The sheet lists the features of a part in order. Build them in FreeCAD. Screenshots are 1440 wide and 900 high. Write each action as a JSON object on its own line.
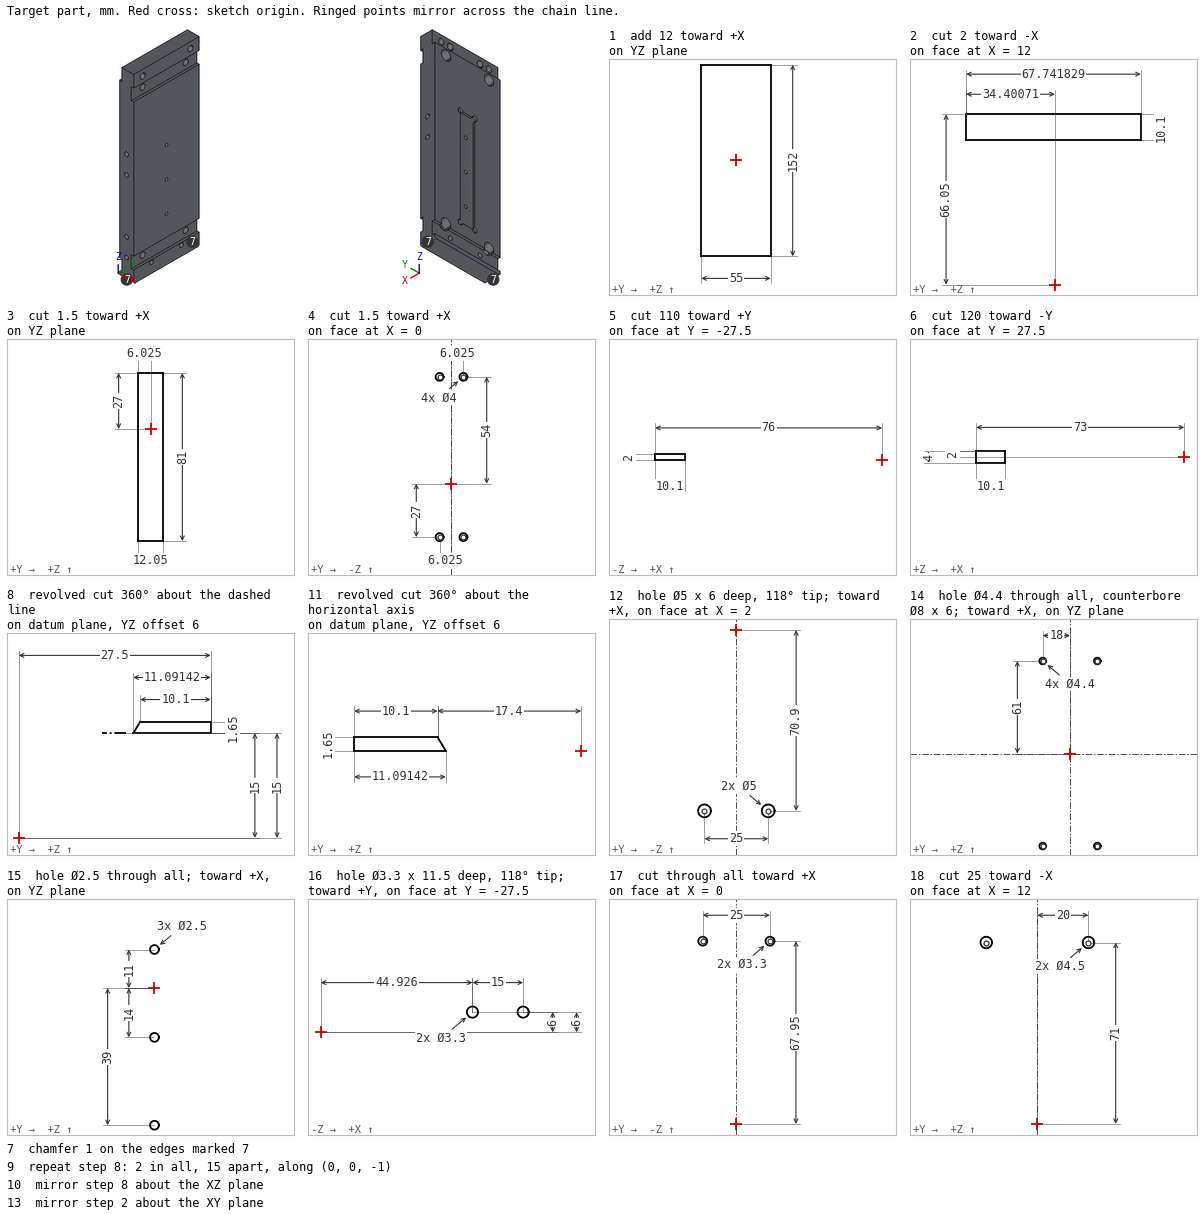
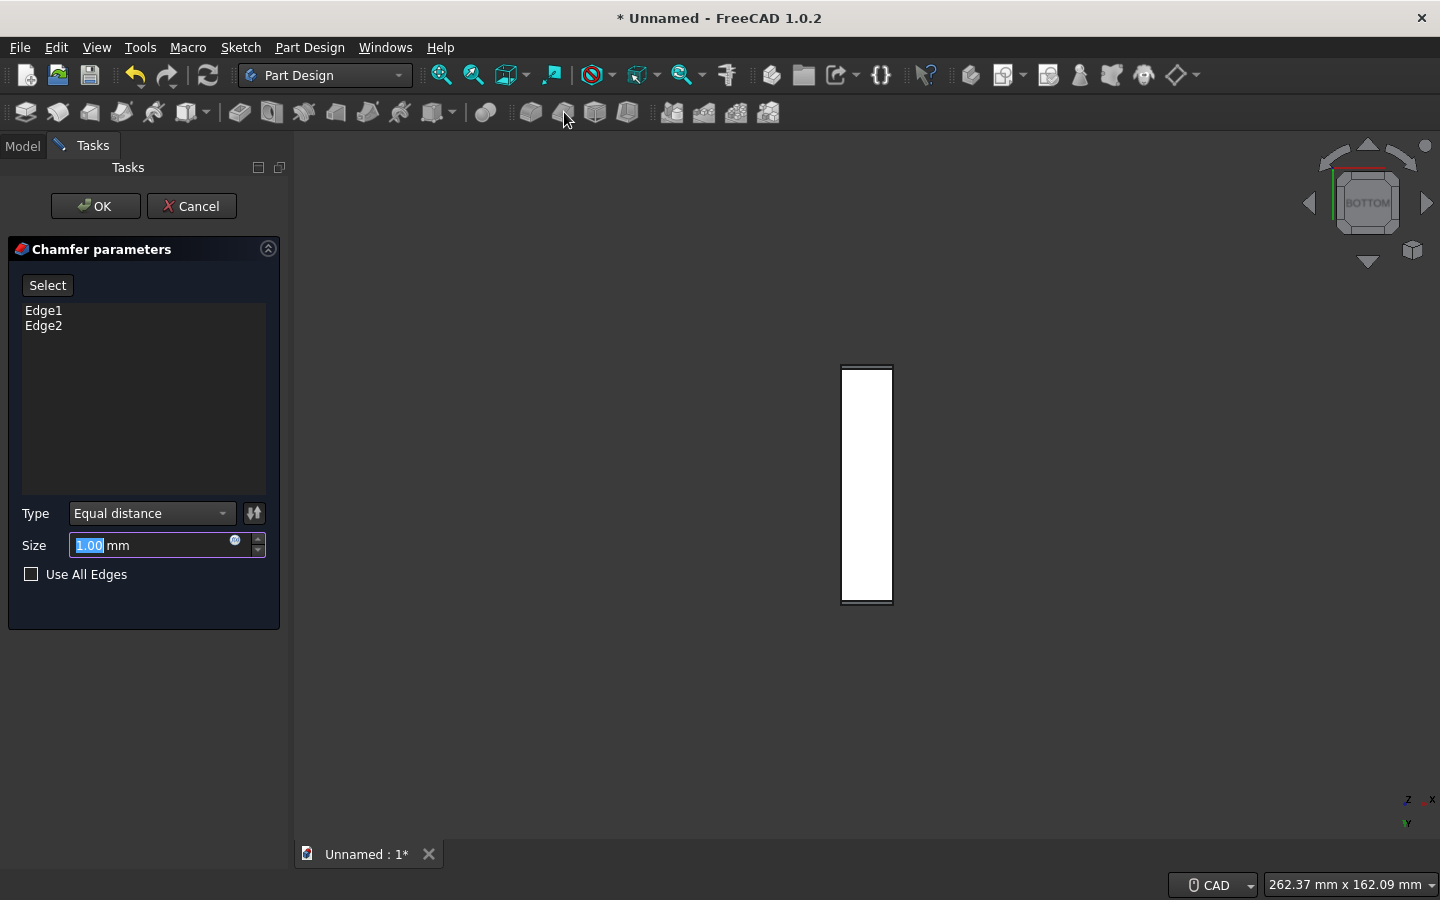
{"action": "type", "text": "1"}
{"action": "key", "text": "Tab"}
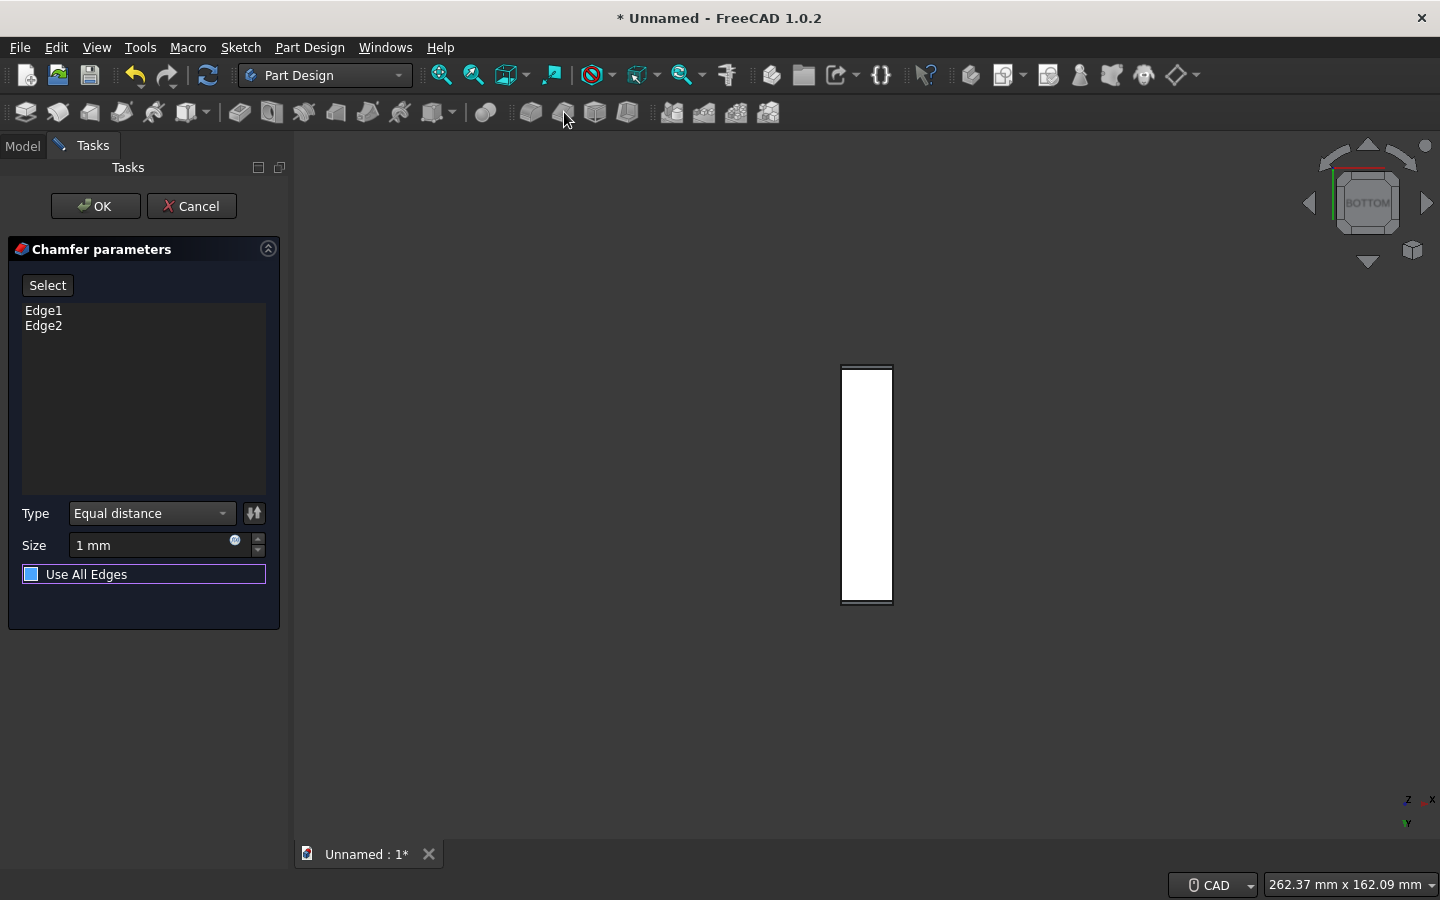
{"action": "left_click", "coordinate": [96, 206]}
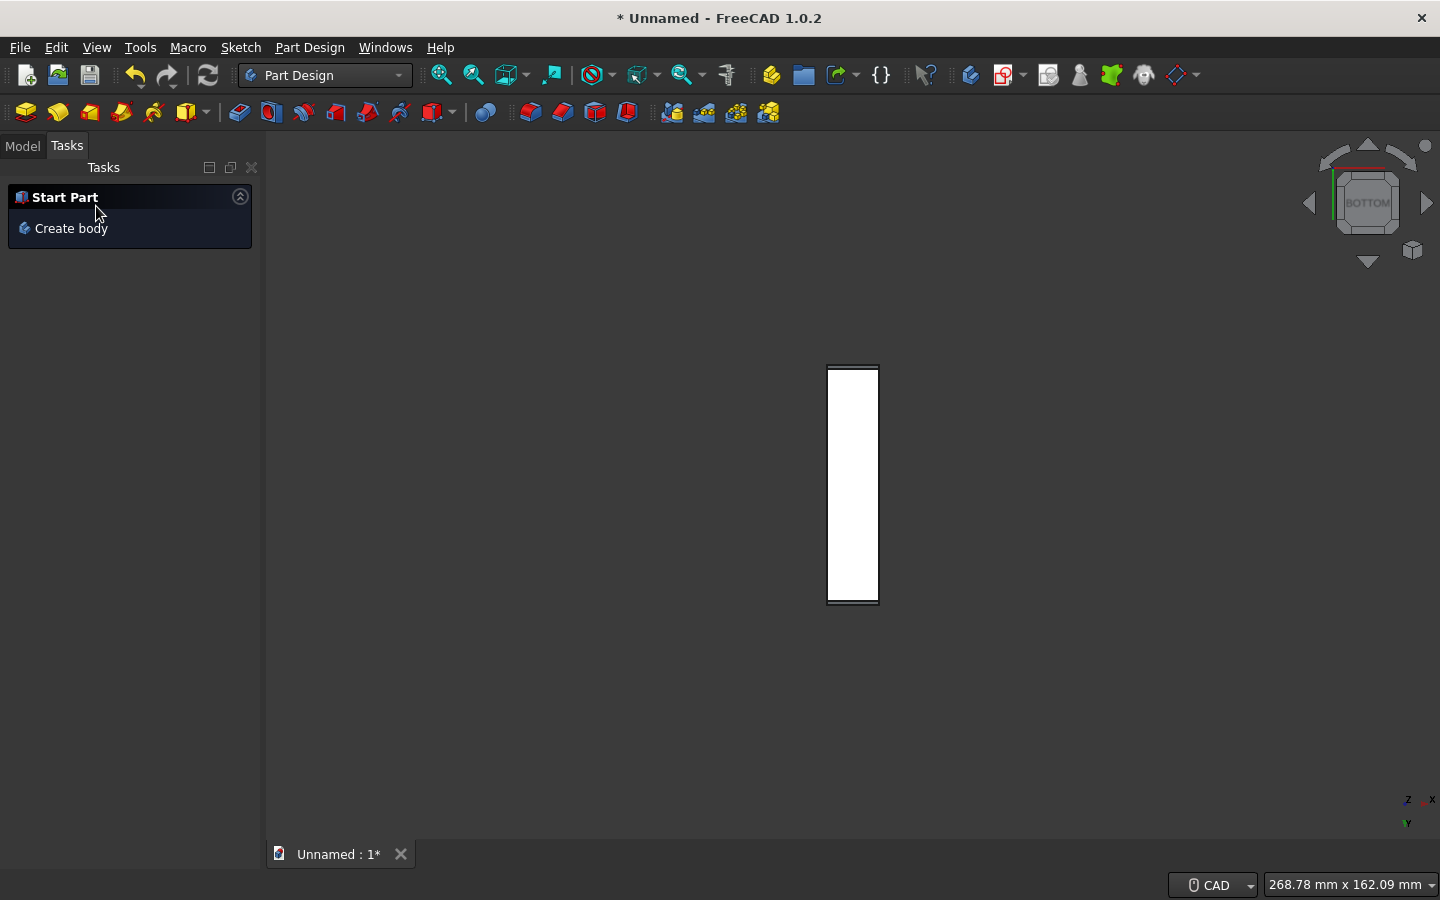
{"action": "left_click", "coordinate": [442, 76]}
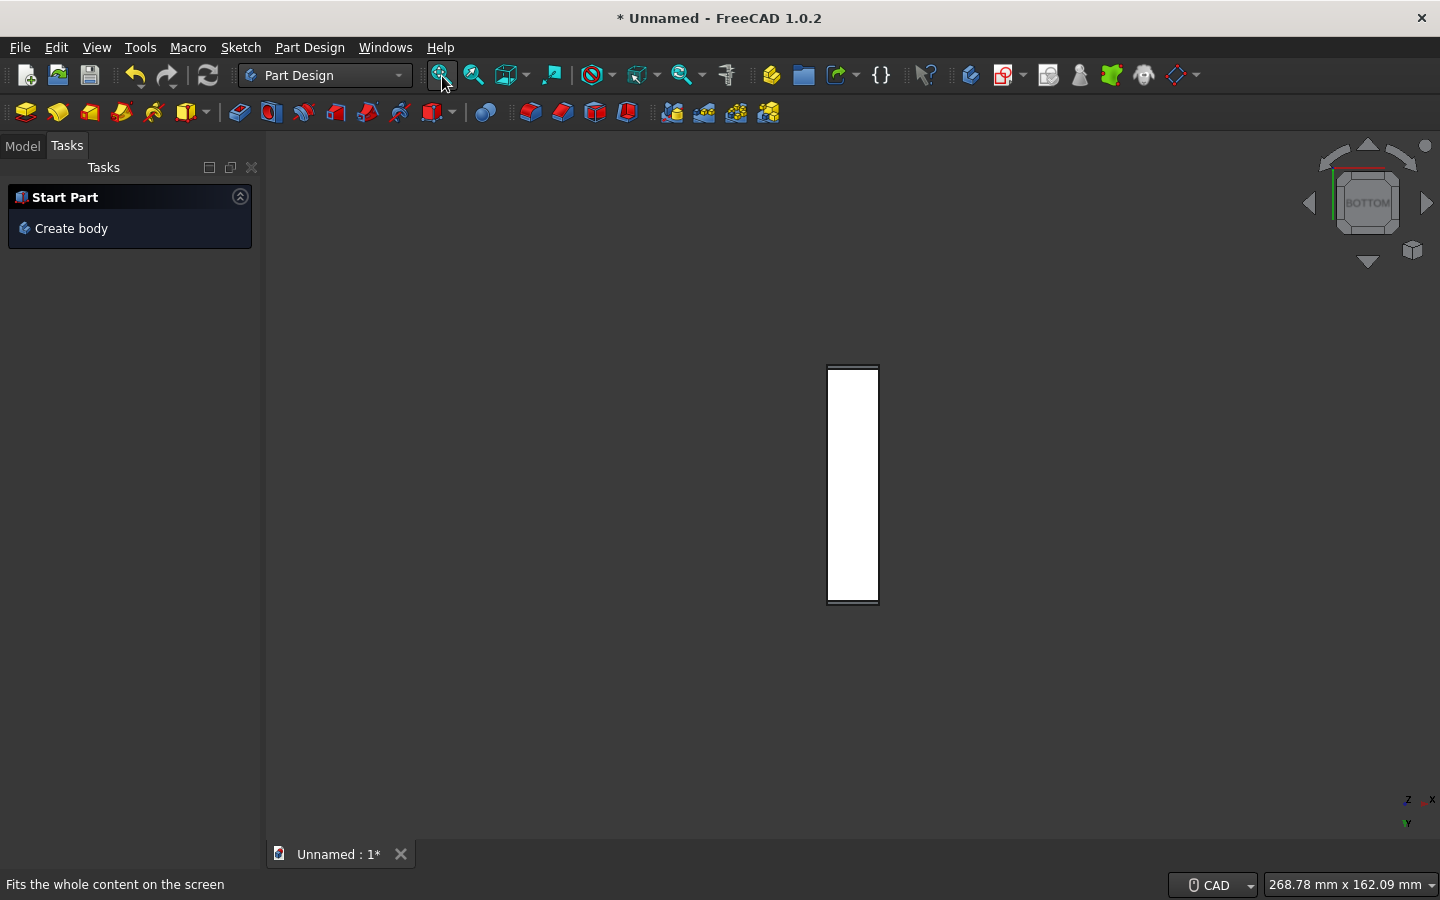
{"action": "left_click", "coordinate": [23, 145]}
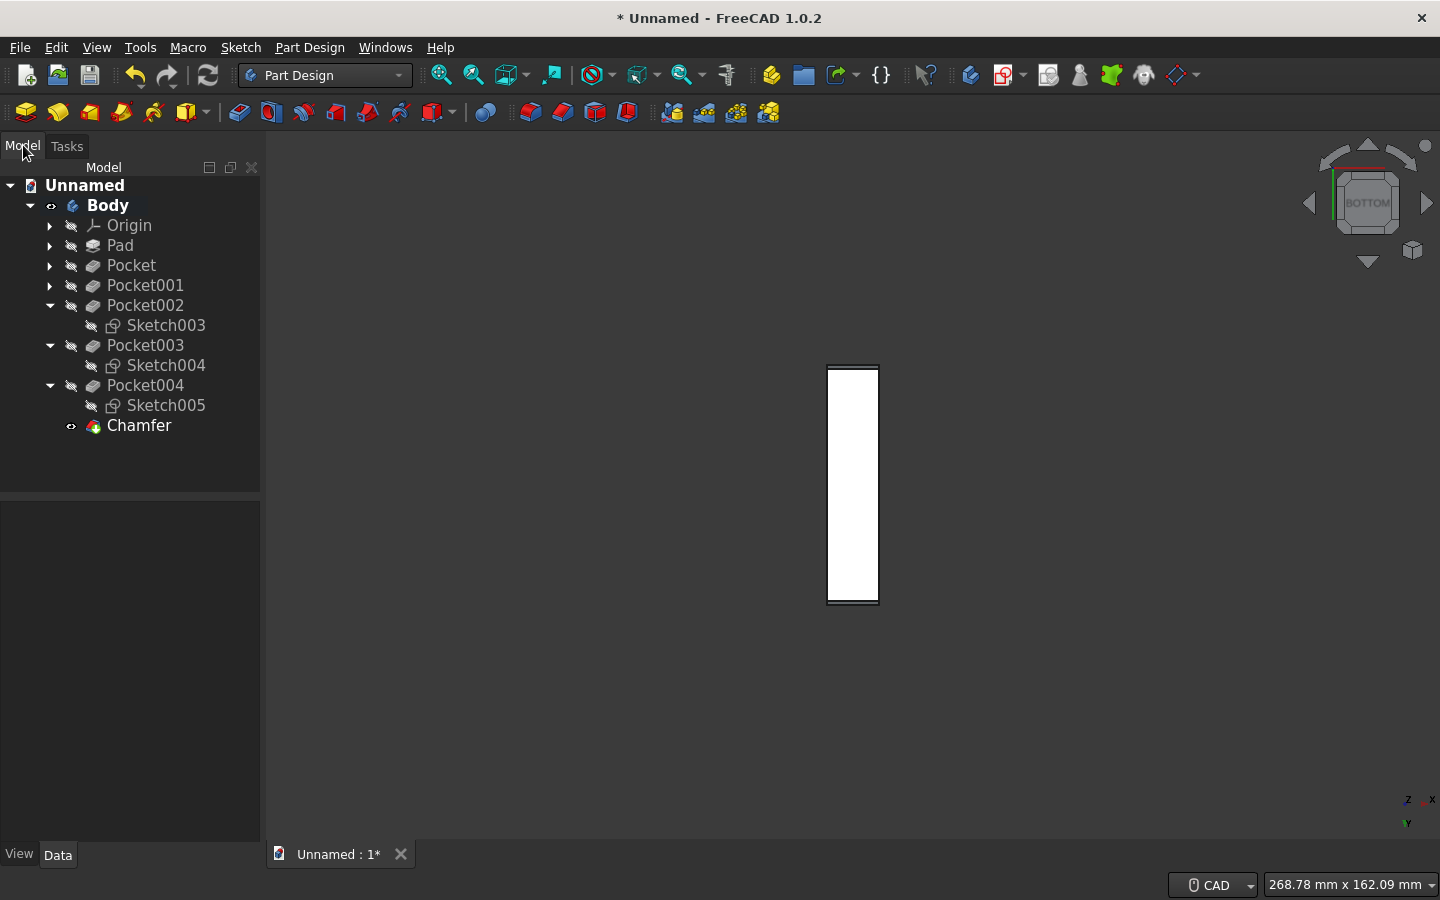
{"action": "left_click", "coordinate": [50, 226]}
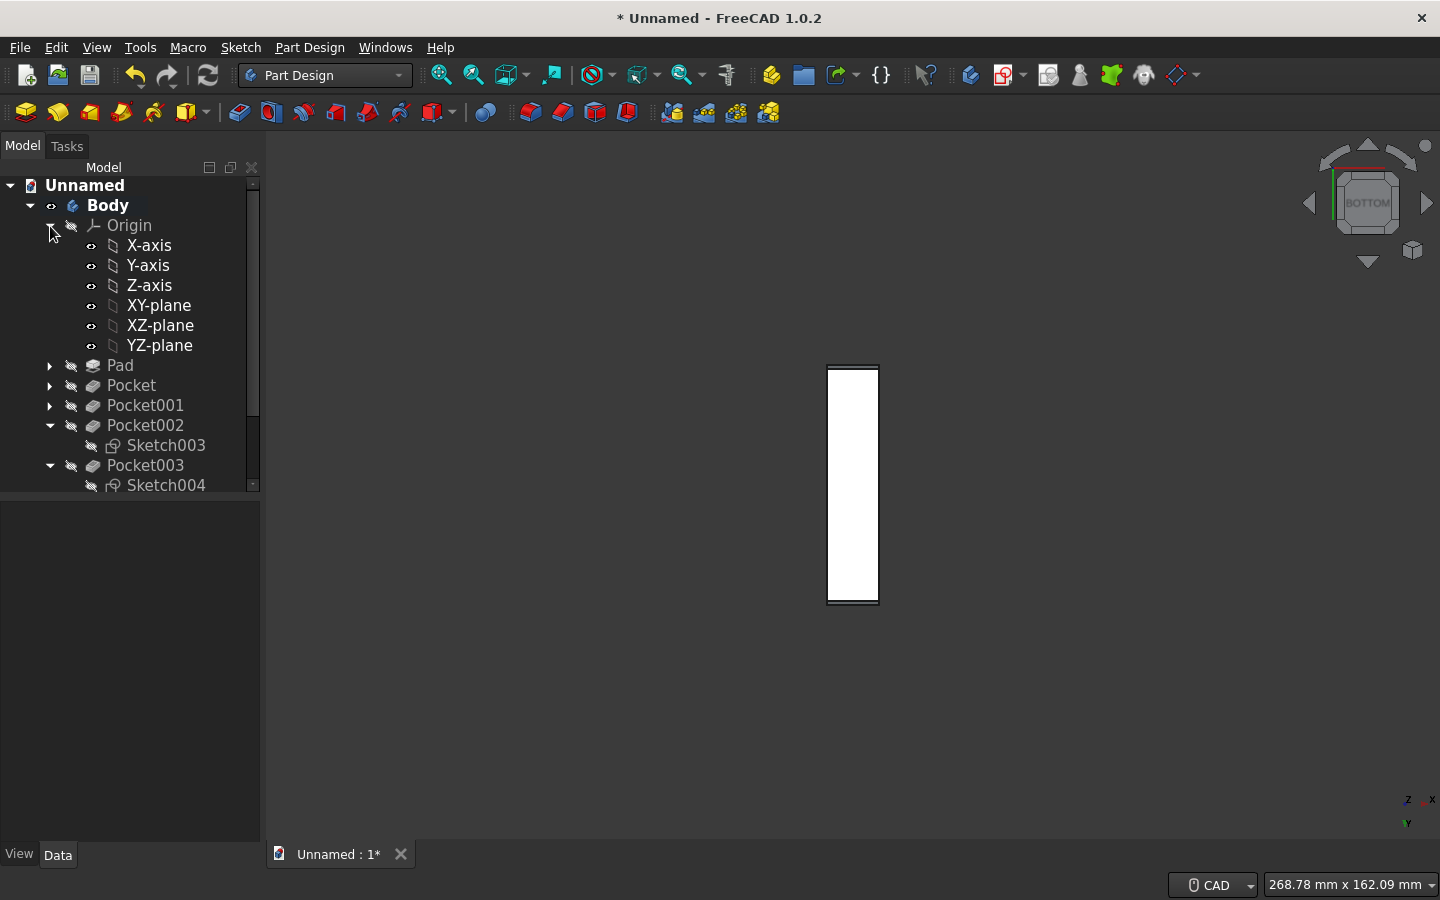
{"action": "left_click", "coordinate": [136, 346]}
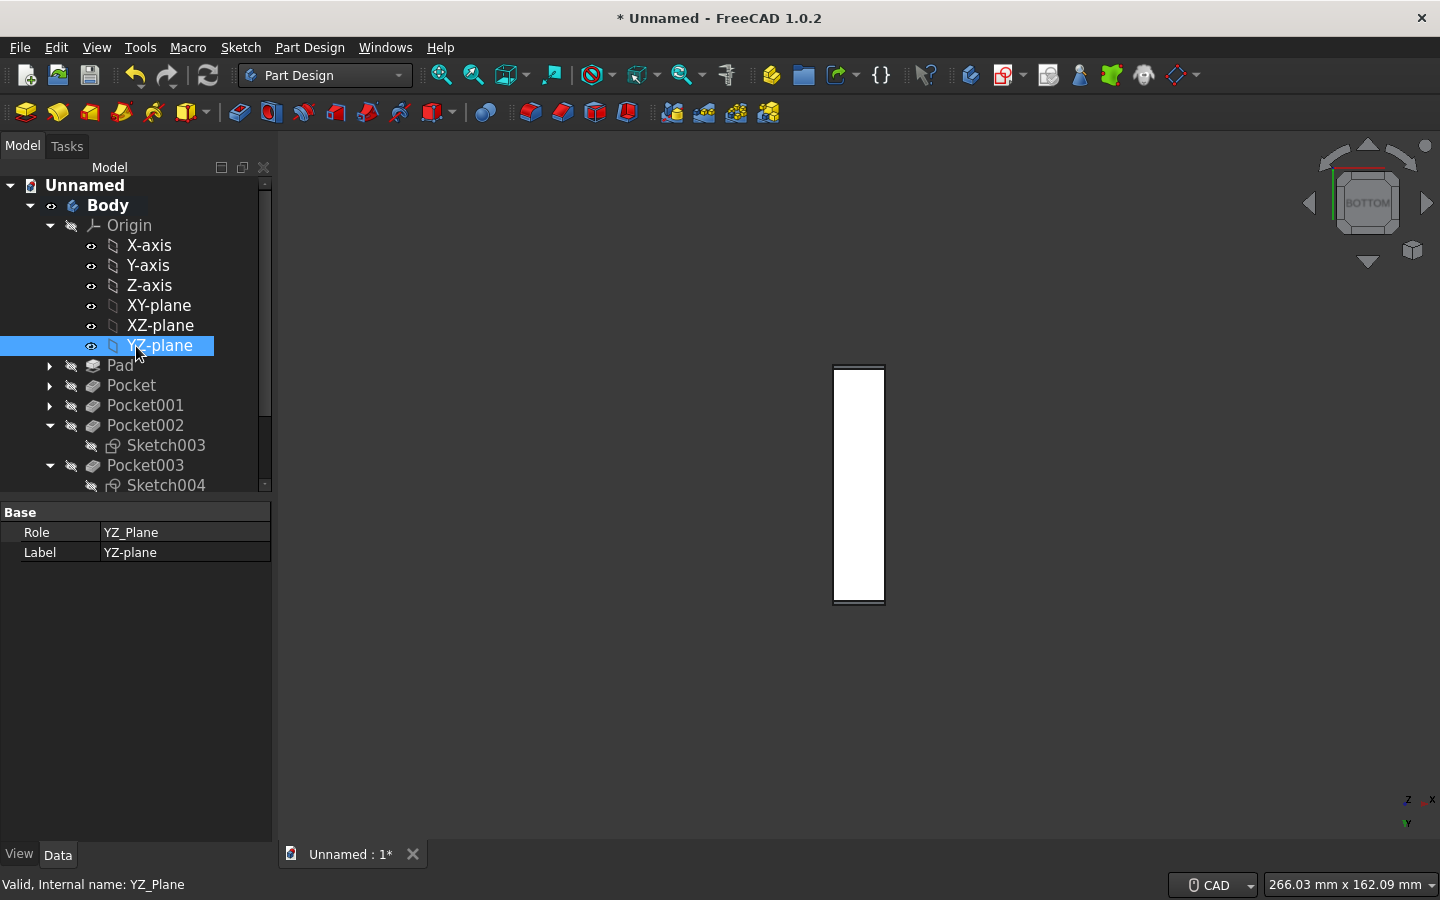
{"action": "left_click", "coordinate": [1176, 76]}